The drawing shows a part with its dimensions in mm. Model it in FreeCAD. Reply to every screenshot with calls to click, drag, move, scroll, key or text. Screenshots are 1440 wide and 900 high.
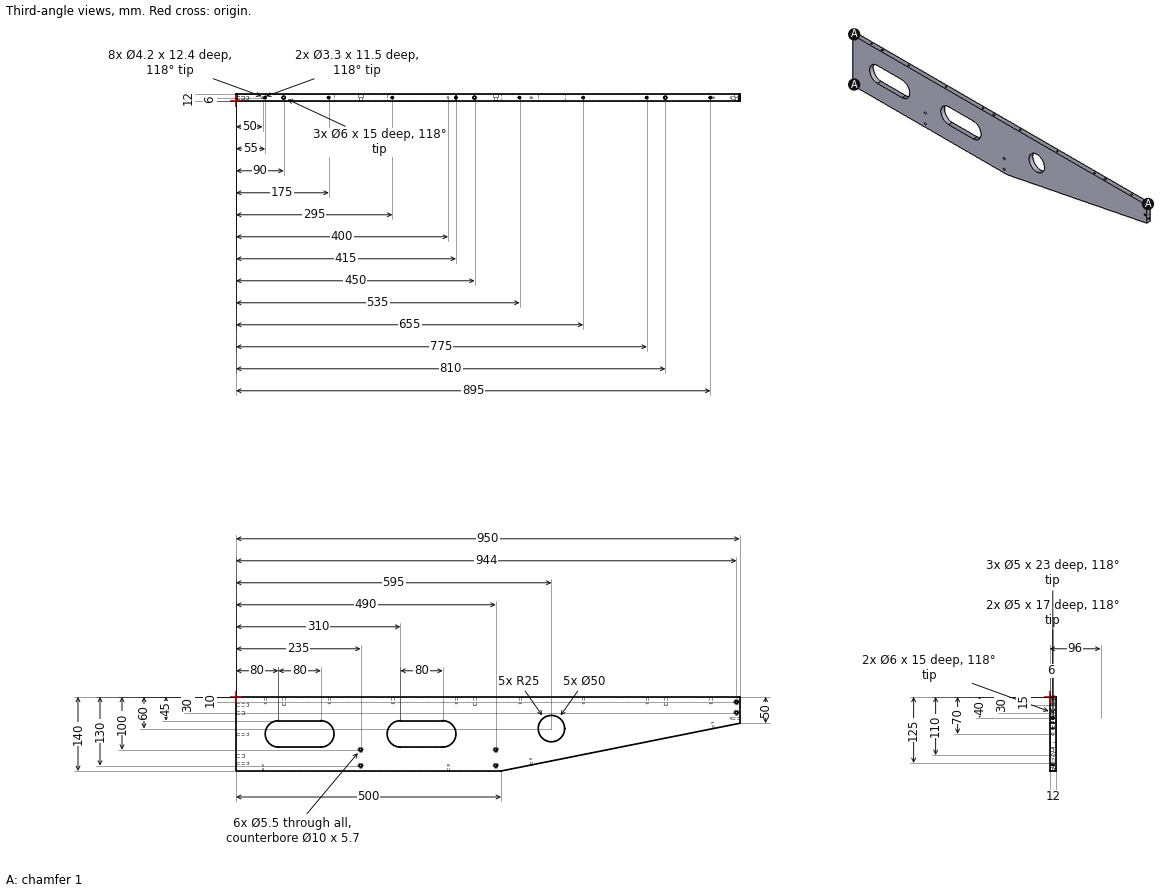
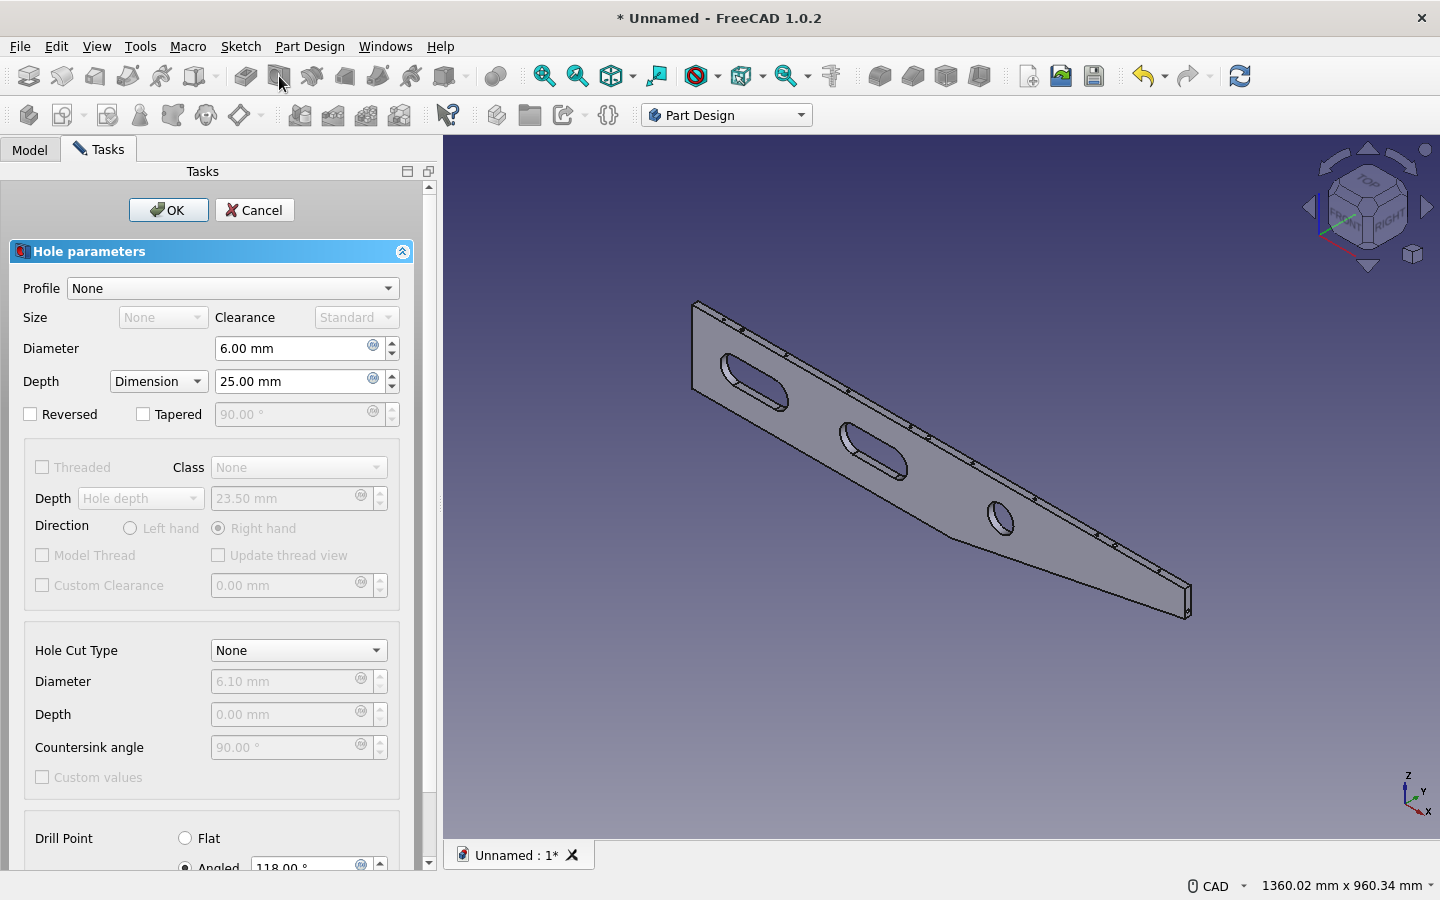
triple_click(300, 348)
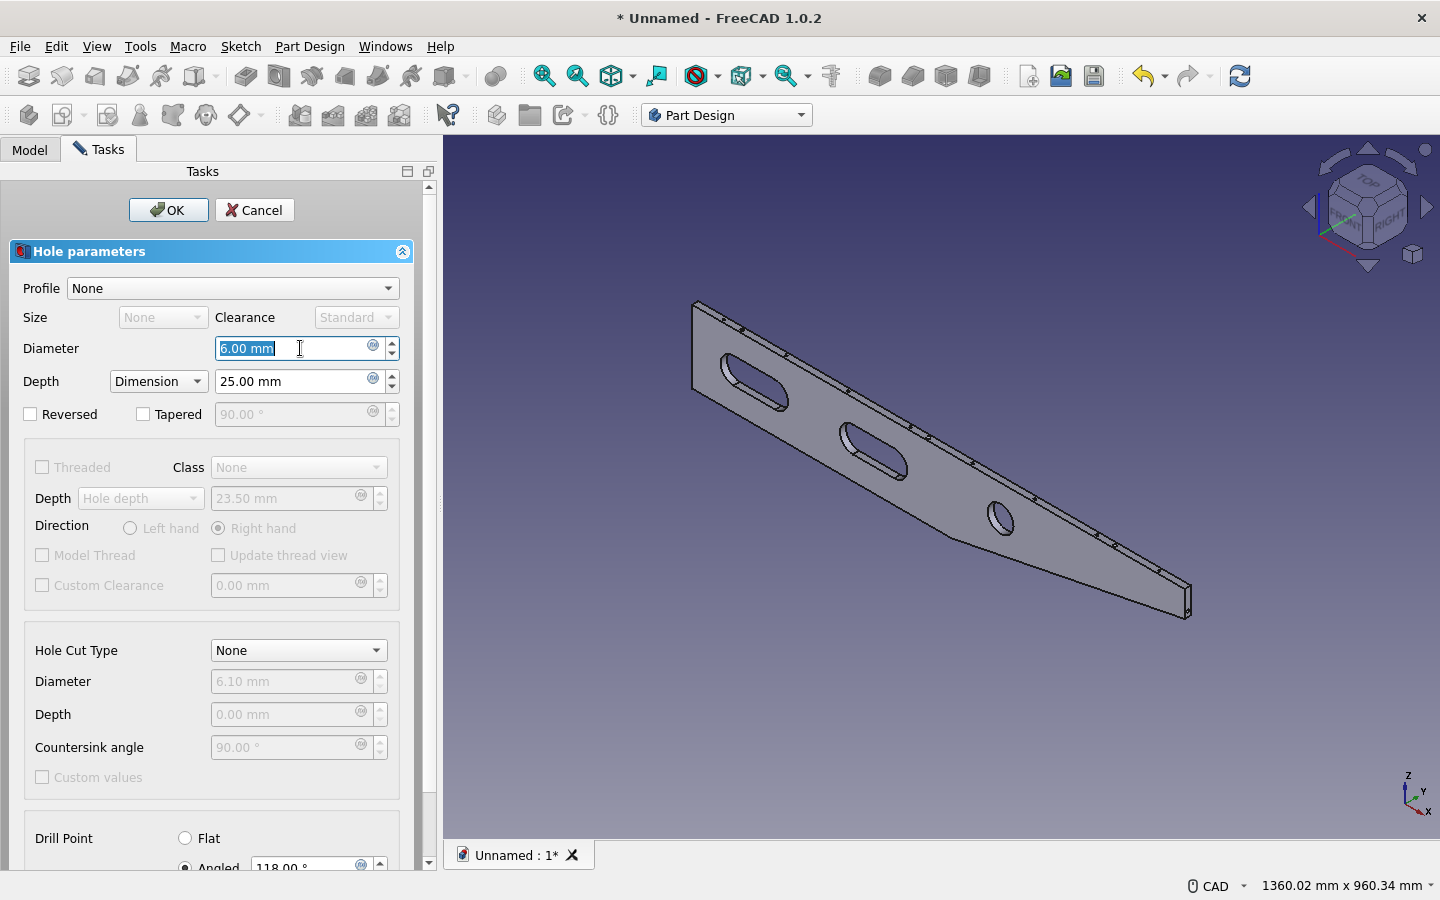
text(6)
key(Tab)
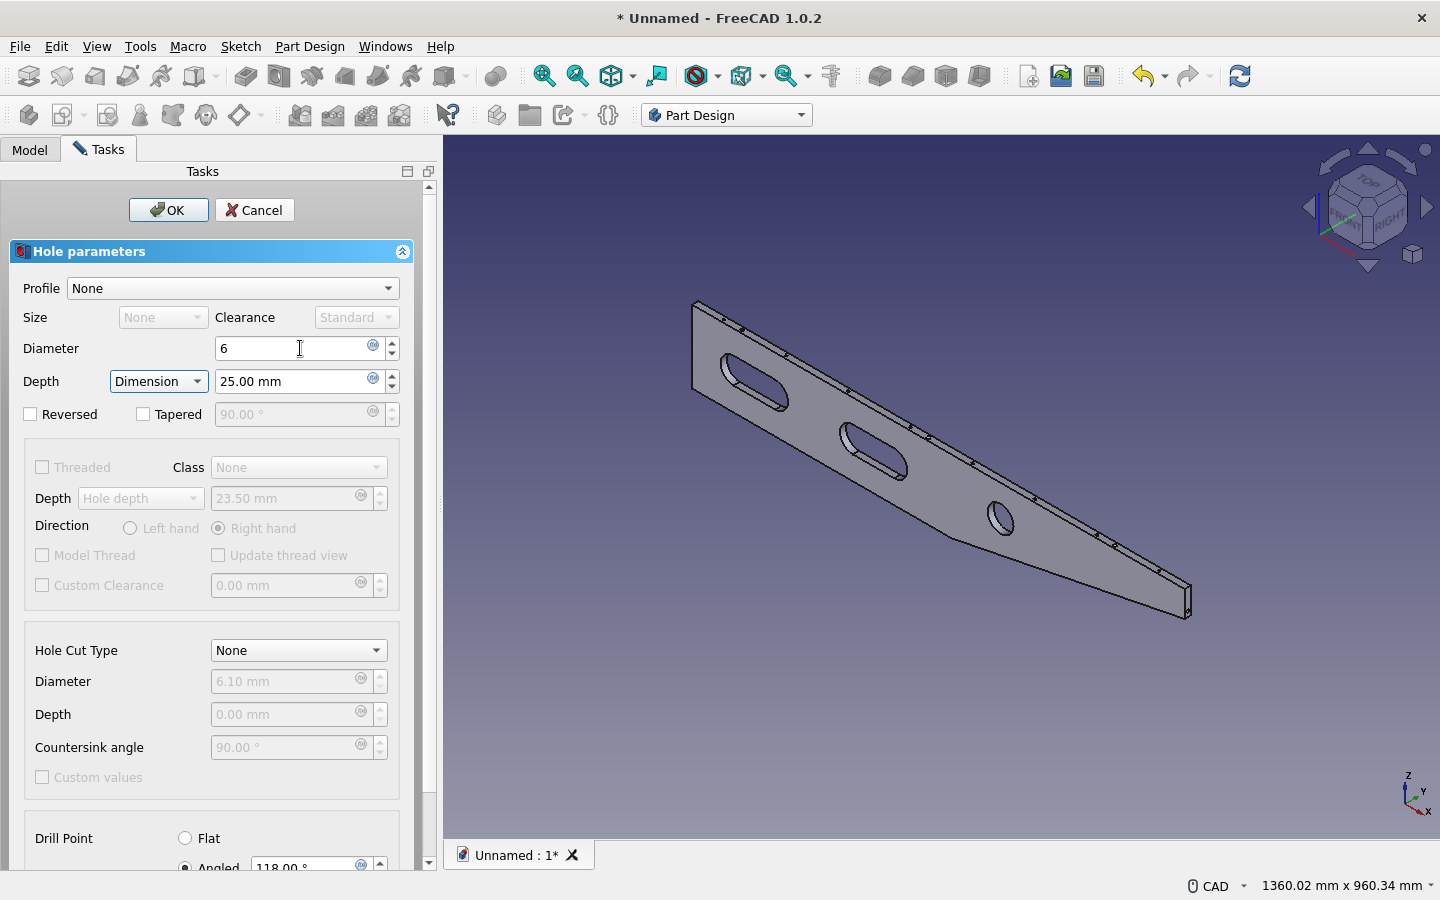
triple_click(300, 382)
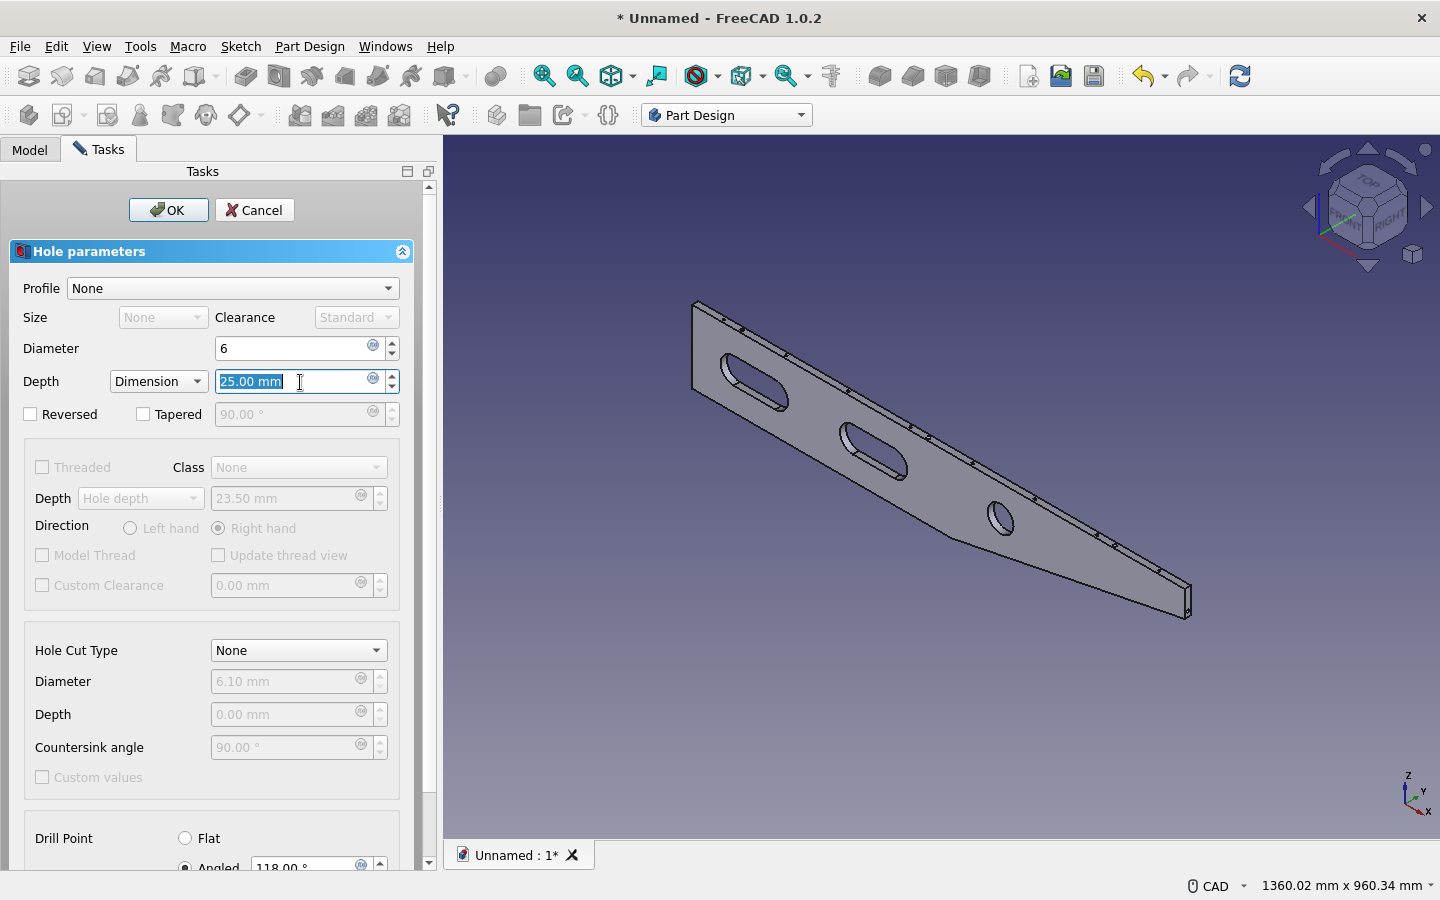
text(15)
key(Tab)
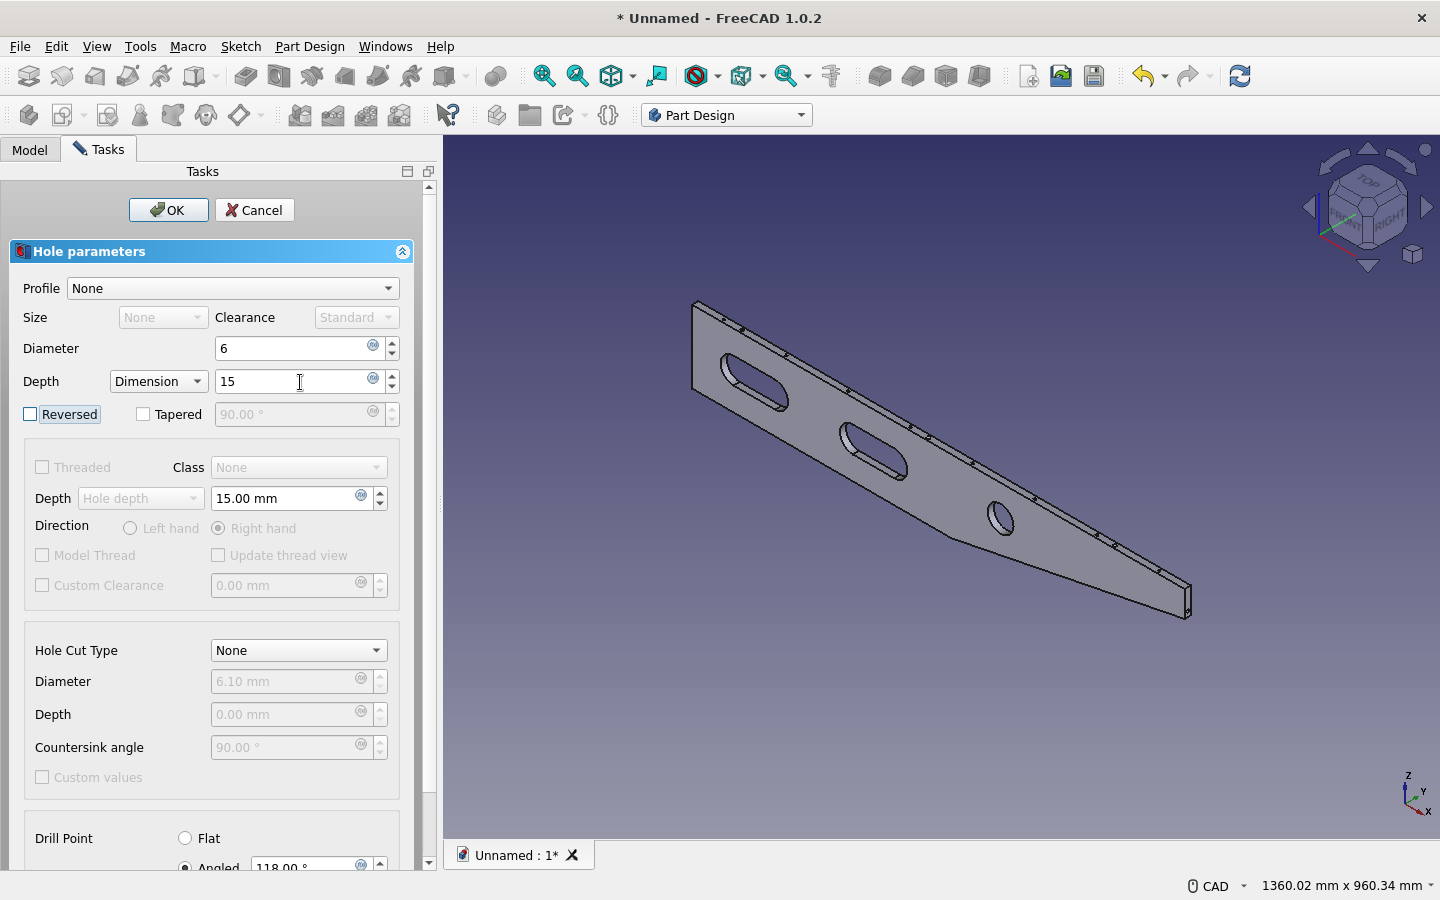
click(169, 210)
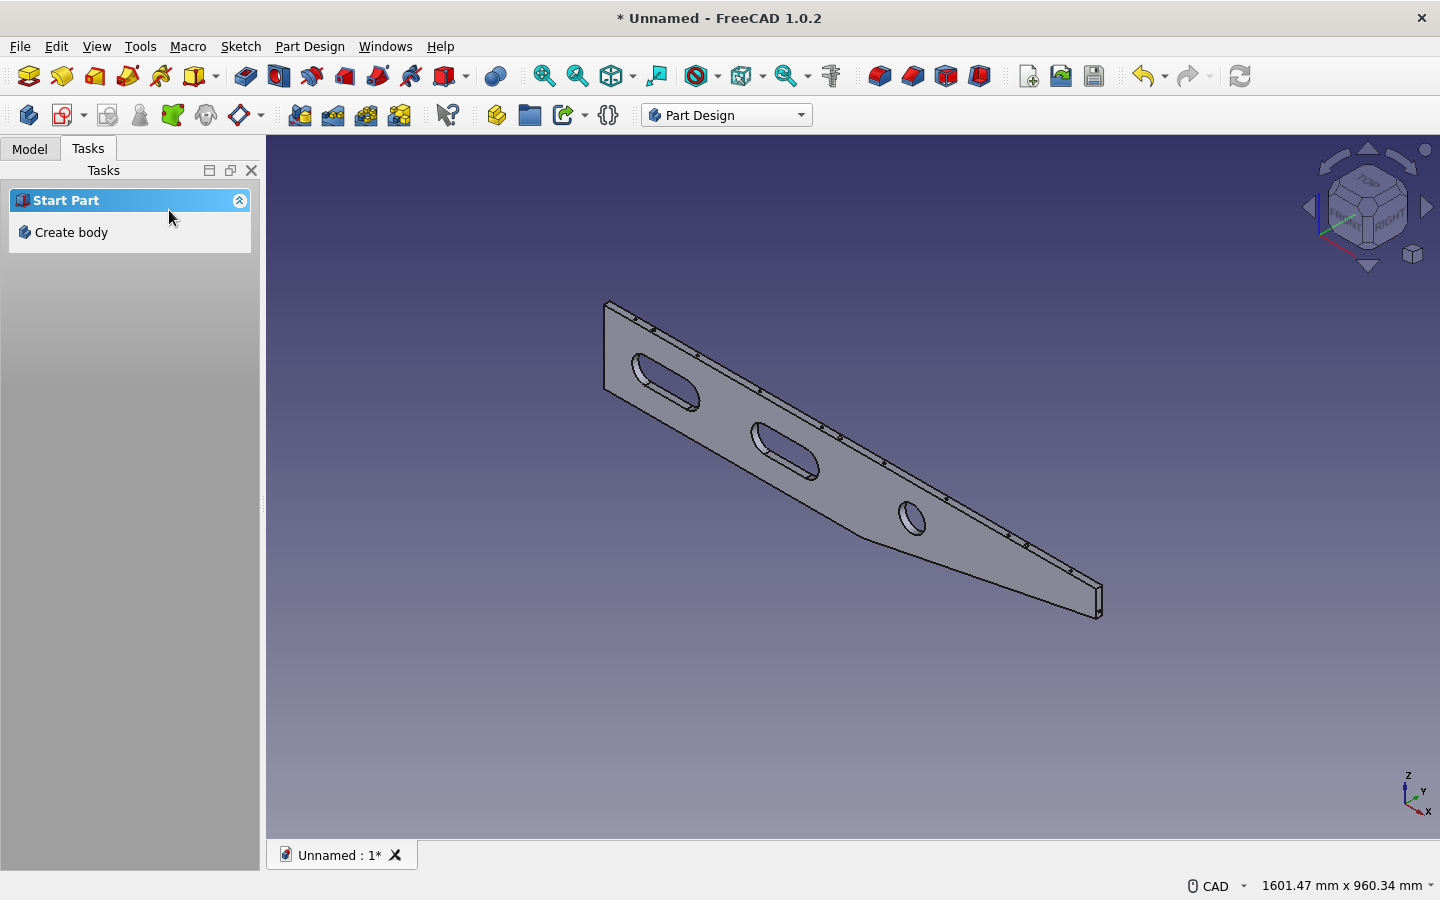
key(4)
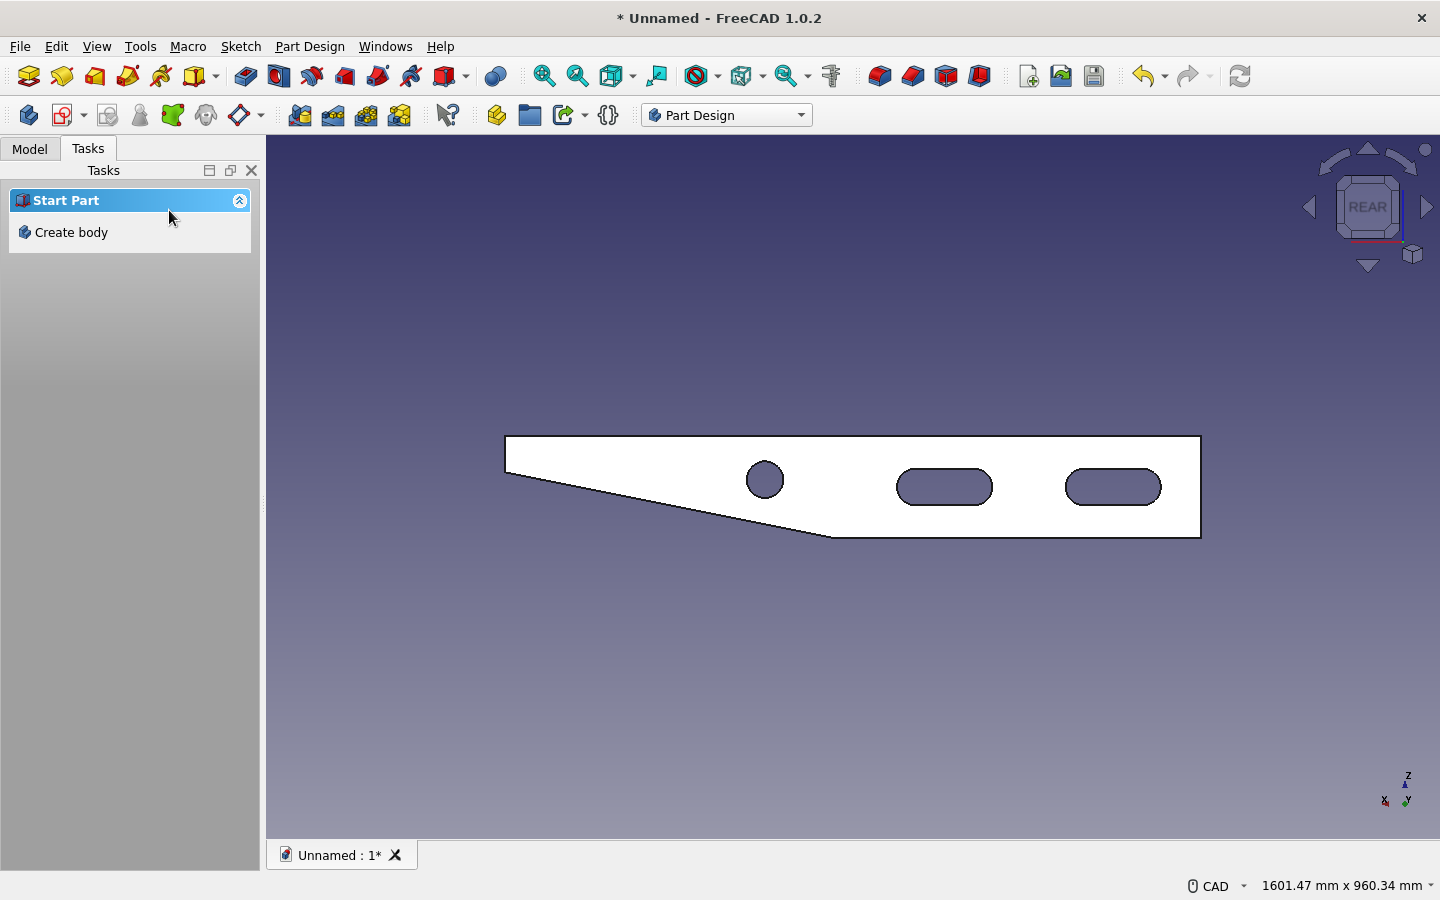
click(853, 486)